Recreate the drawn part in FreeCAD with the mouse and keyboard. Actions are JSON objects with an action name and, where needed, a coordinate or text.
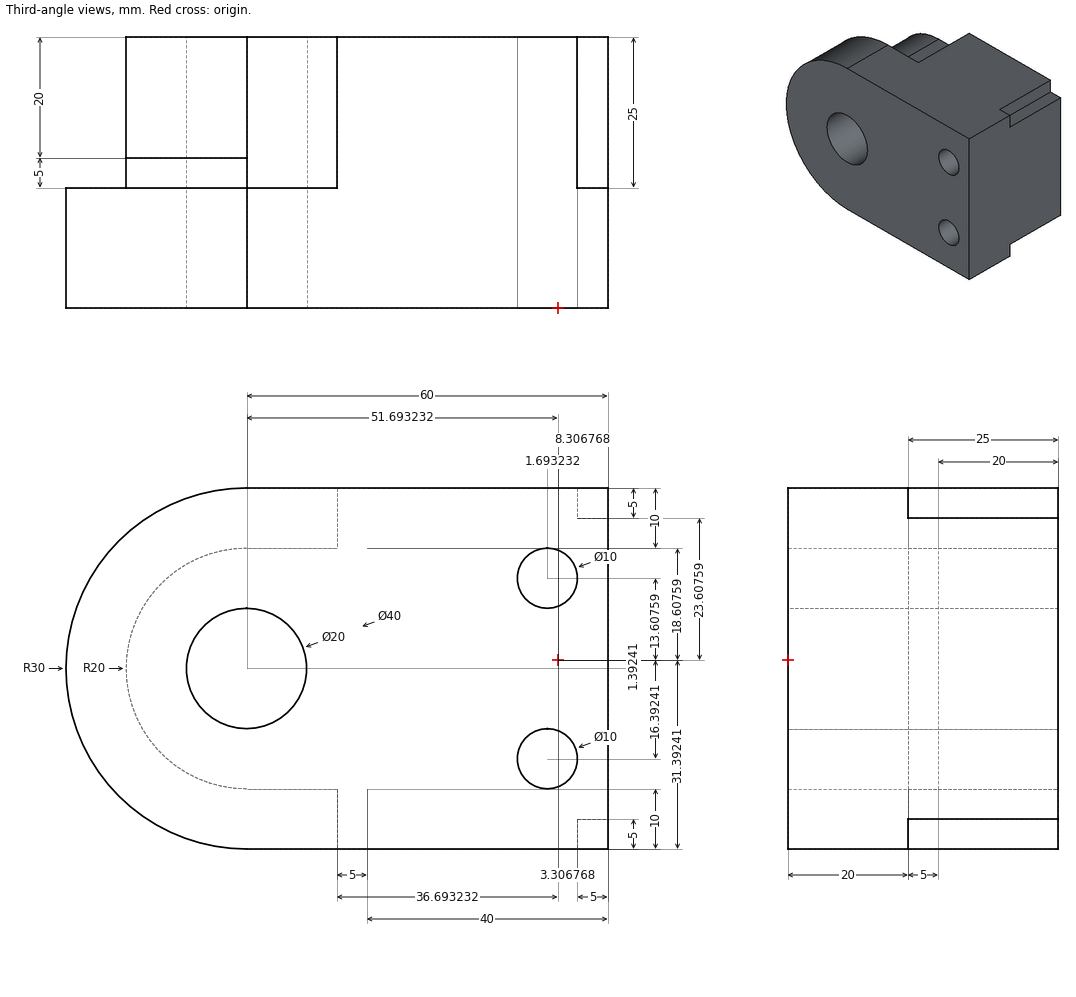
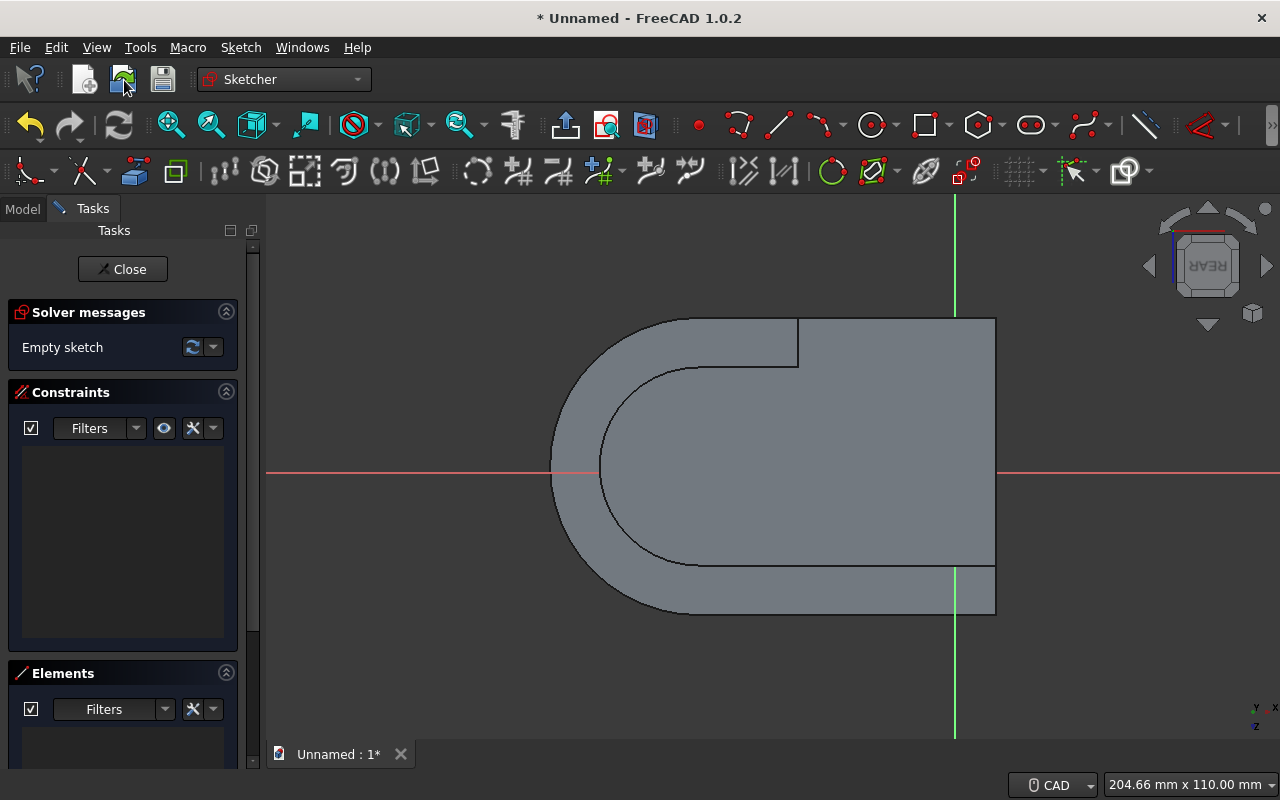
{"action": "key", "text": "q s"}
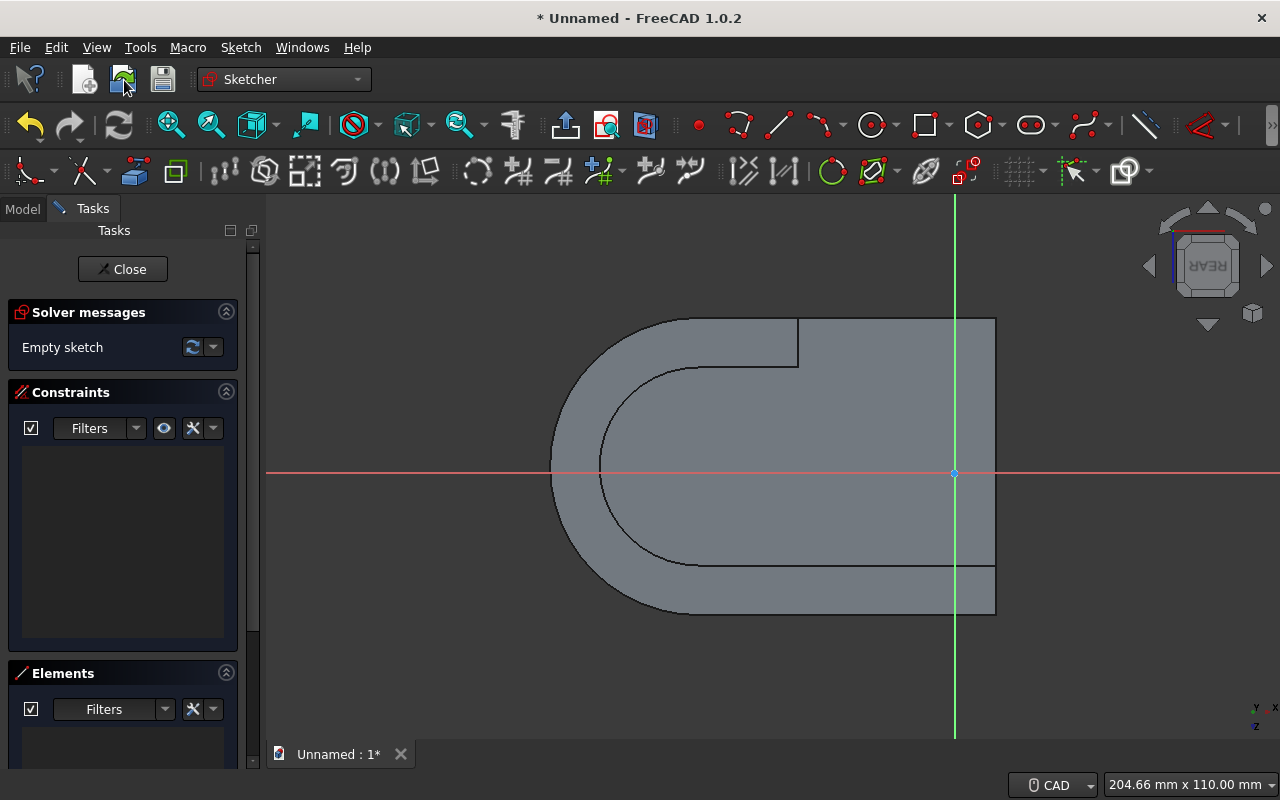
{"action": "scroll", "coordinate": [1054, 608], "scroll_direction": "up", "scroll_amount": 4}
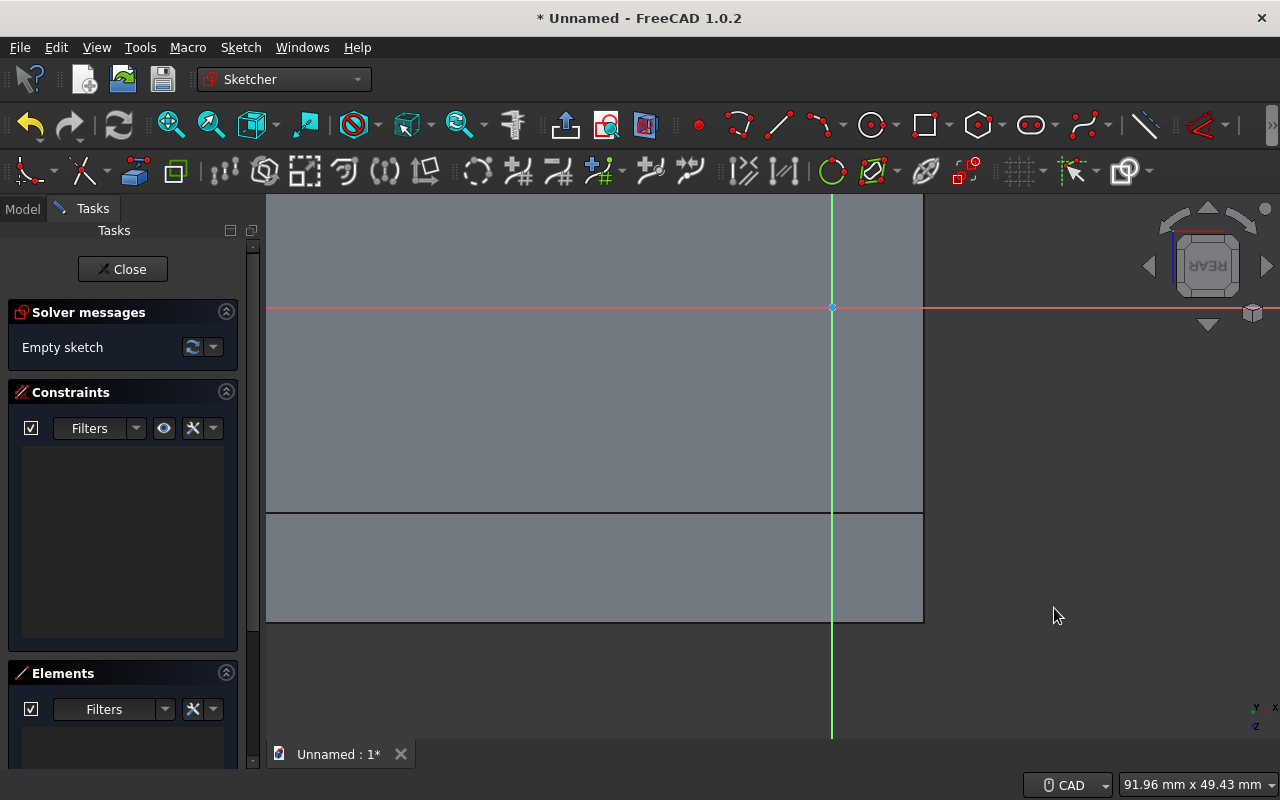
{"action": "left_click", "coordinate": [926, 126]}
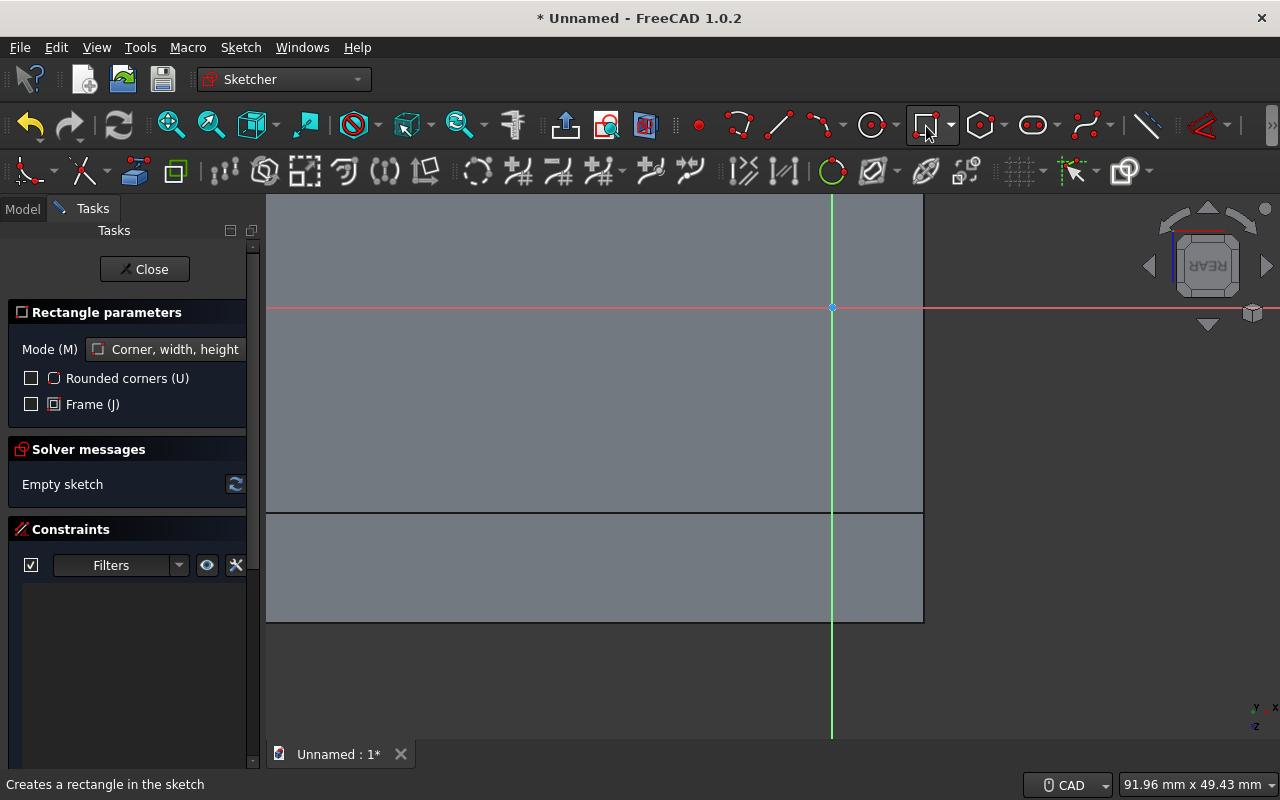
{"action": "left_click", "coordinate": [483, 513]}
{"action": "left_click", "coordinate": [924, 623]}
{"action": "key", "text": "Escape"}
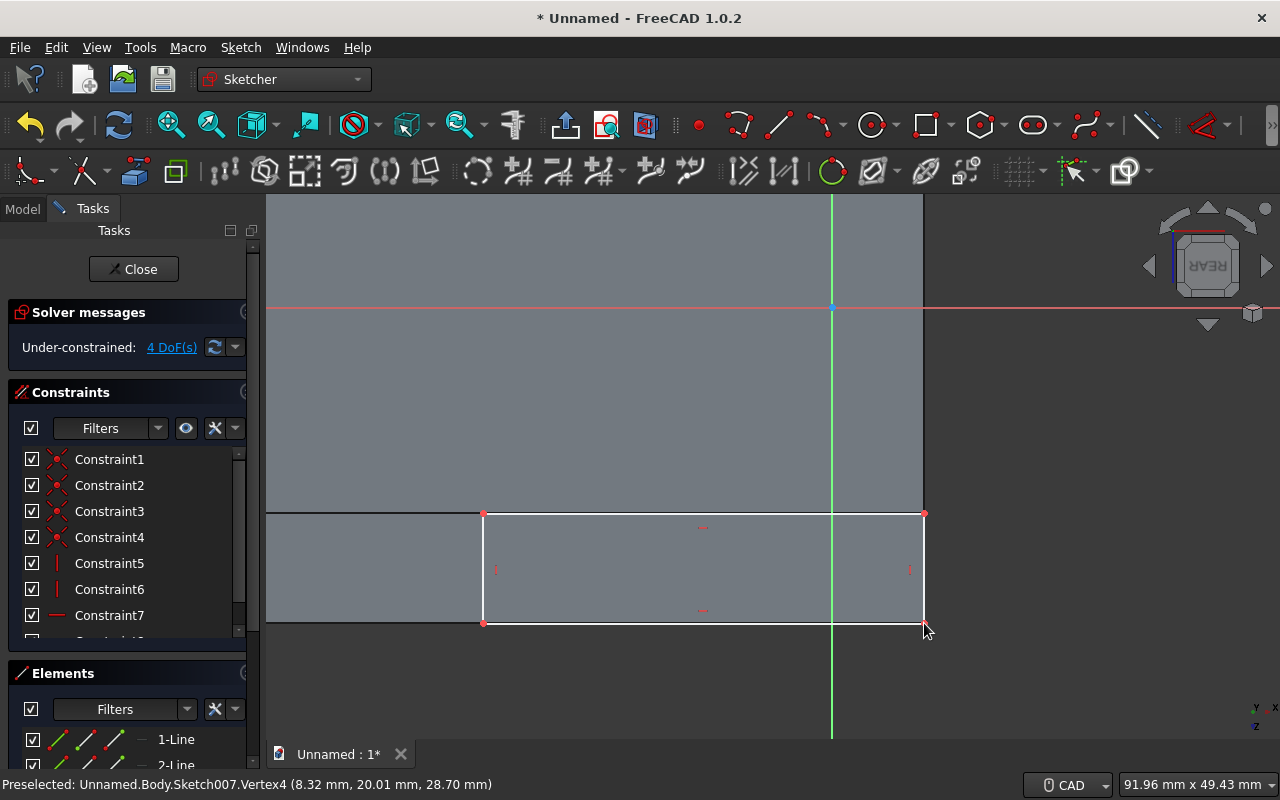
{"action": "key", "text": "d"}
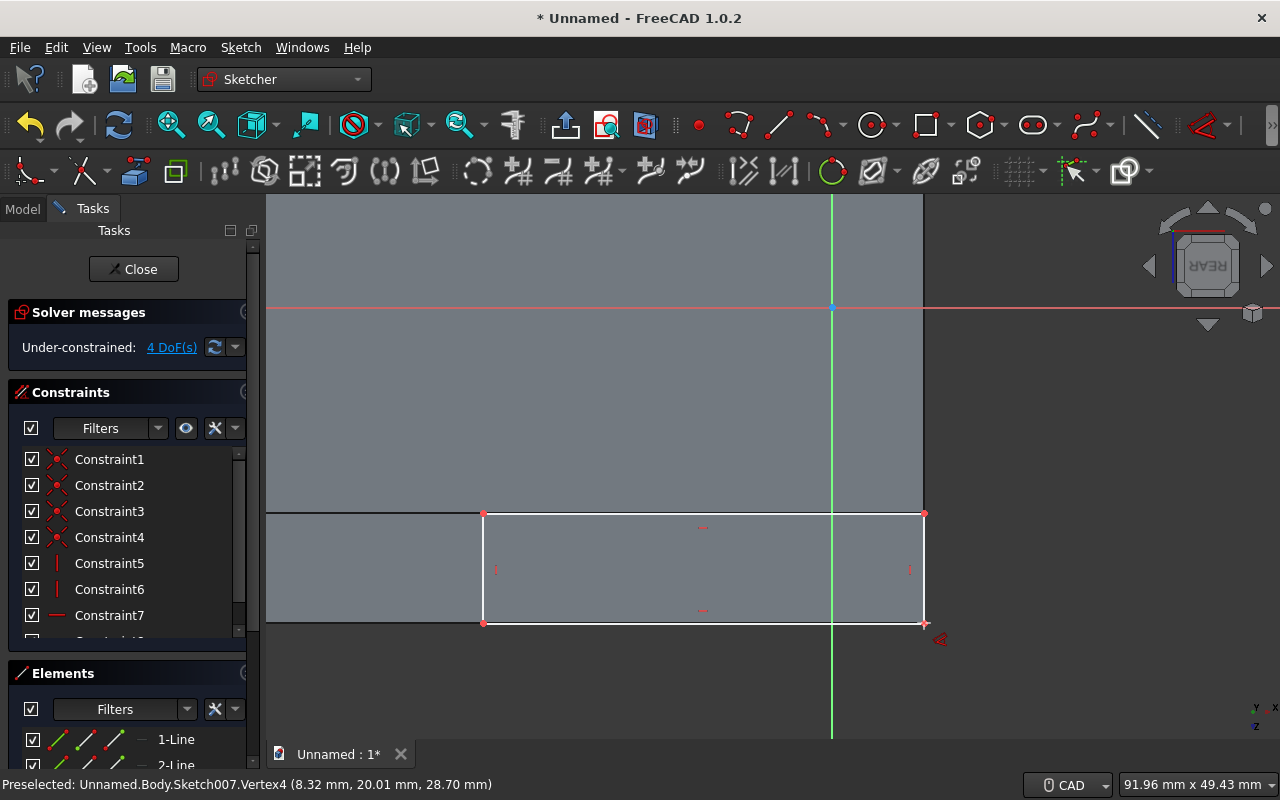
{"action": "left_click", "coordinate": [483, 547]}
{"action": "left_click", "coordinate": [449, 569]}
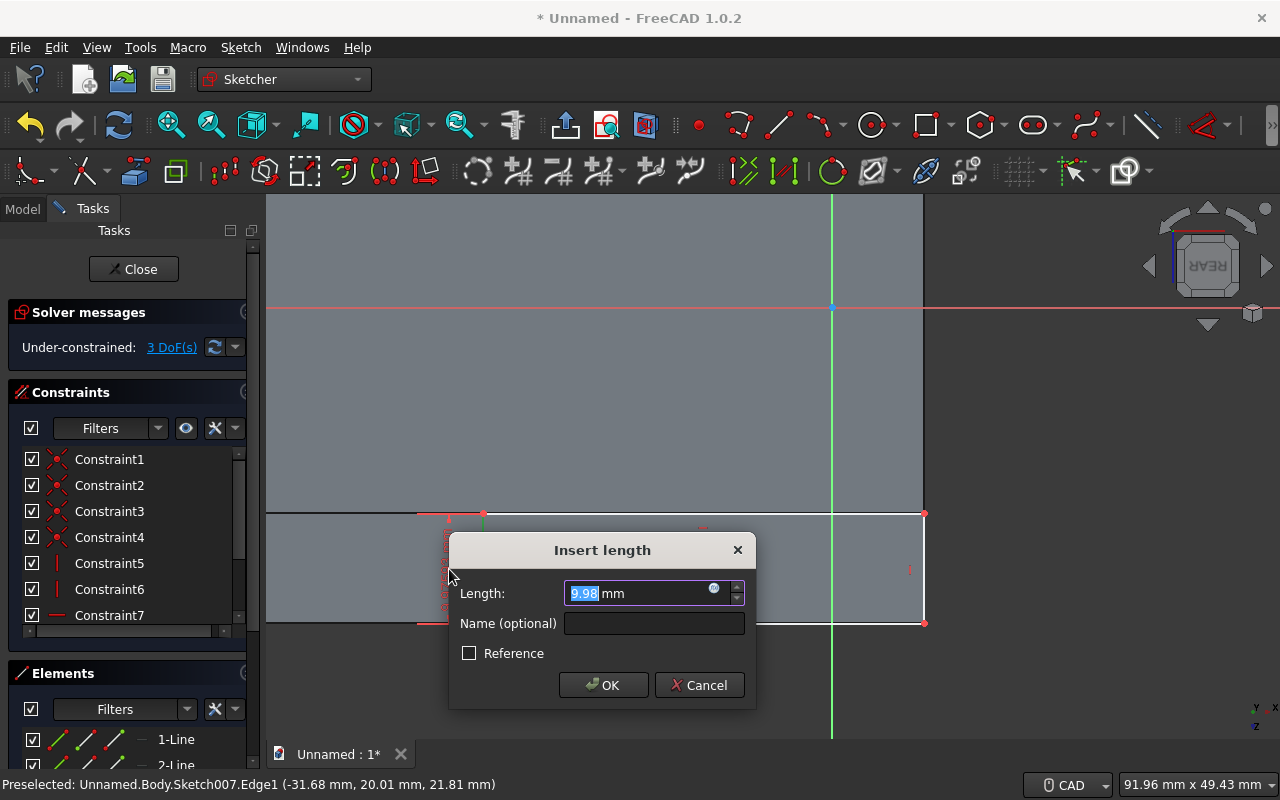
{"action": "type", "text": "10"}
{"action": "key", "text": "Return"}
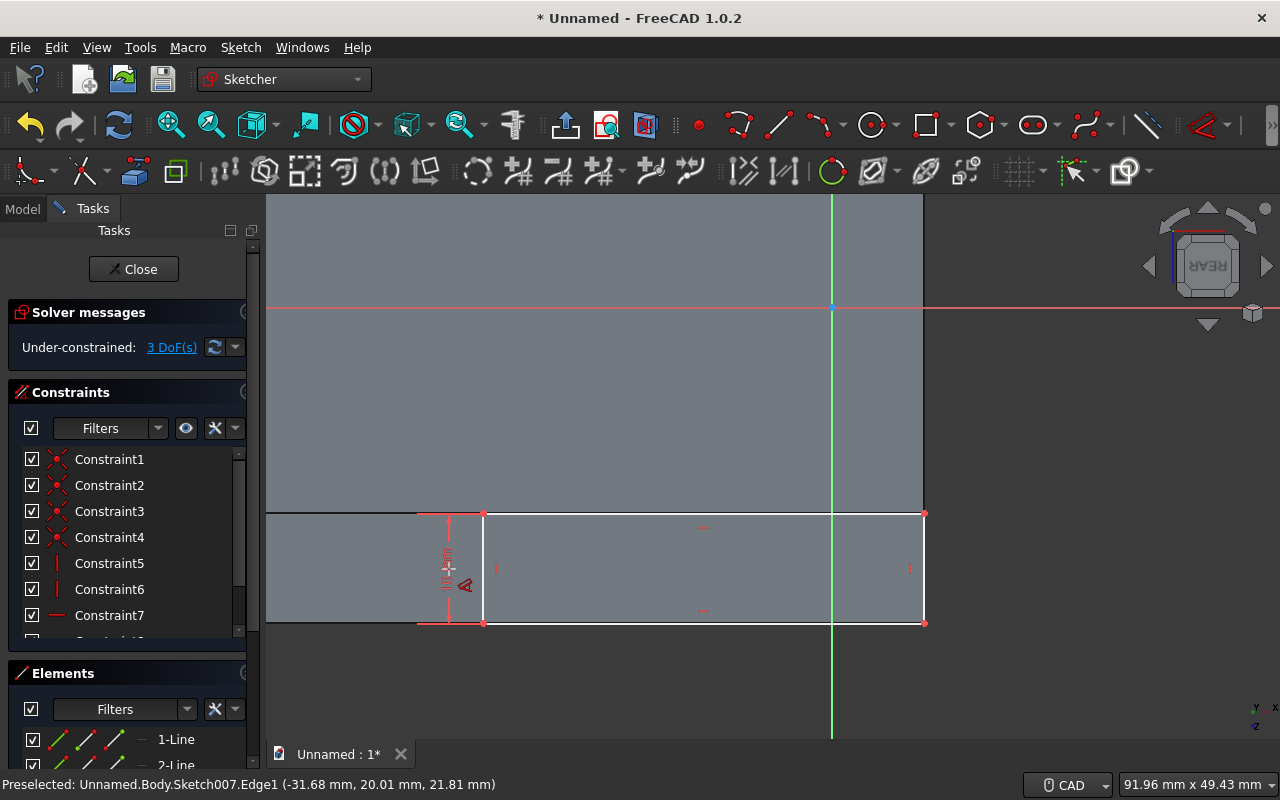
{"action": "left_click", "coordinate": [615, 624]}
{"action": "left_click", "coordinate": [703, 658]}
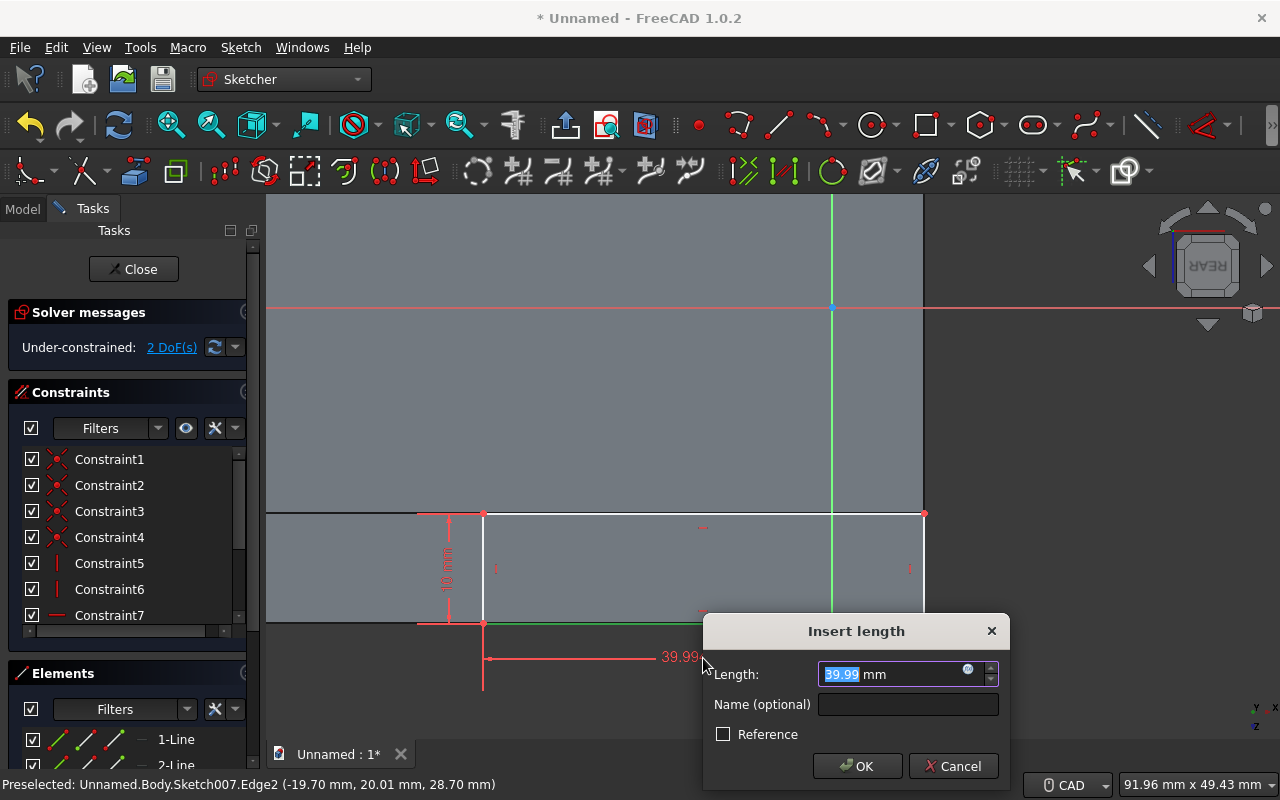
{"action": "type", "text": "40"}
{"action": "key", "text": "Return"}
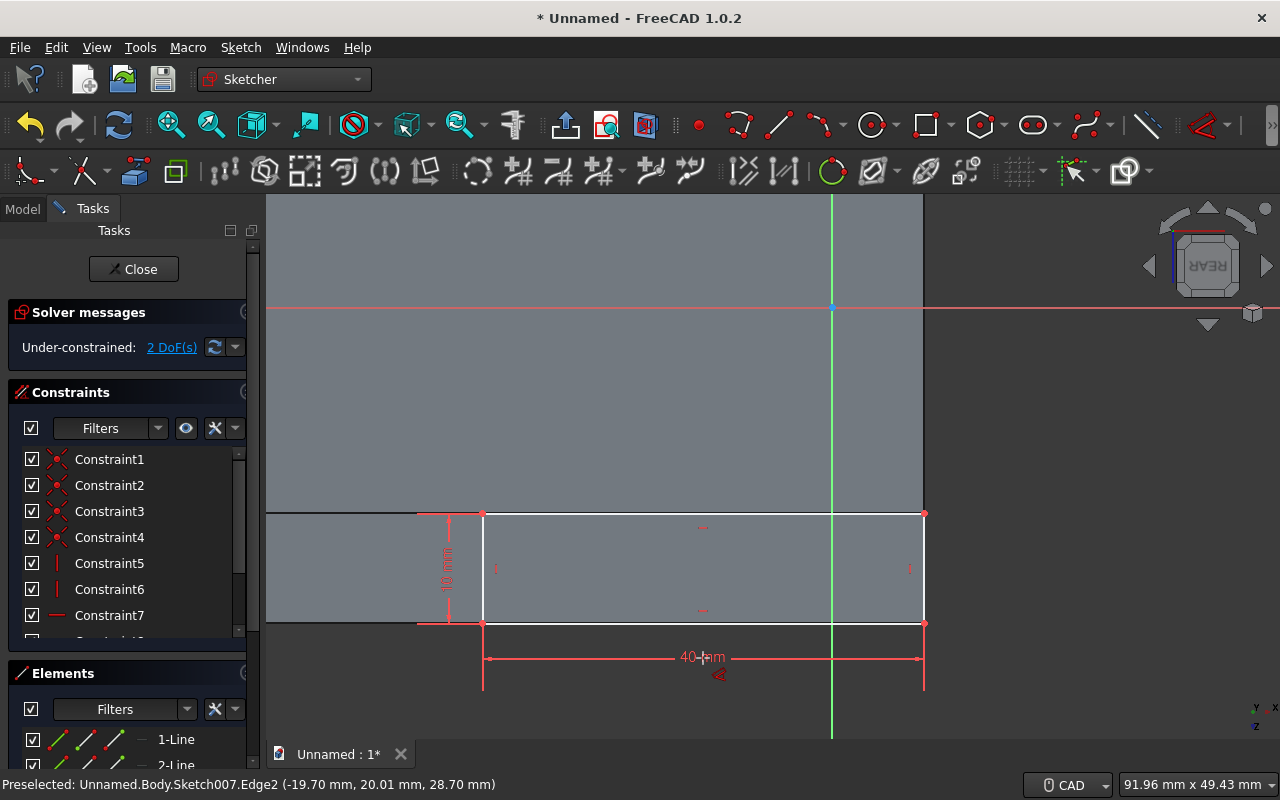
{"action": "left_click", "coordinate": [483, 514]}
{"action": "left_click", "coordinate": [449, 411]}